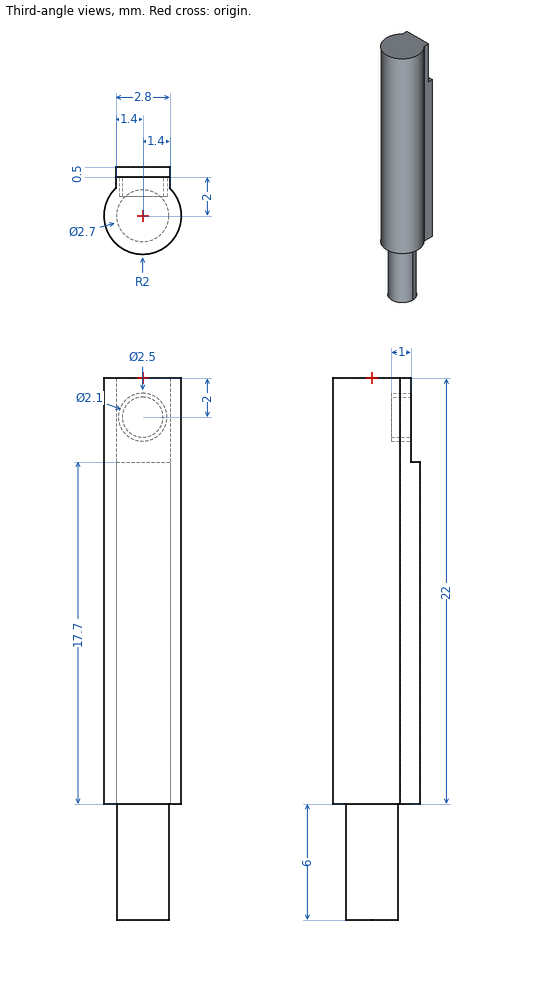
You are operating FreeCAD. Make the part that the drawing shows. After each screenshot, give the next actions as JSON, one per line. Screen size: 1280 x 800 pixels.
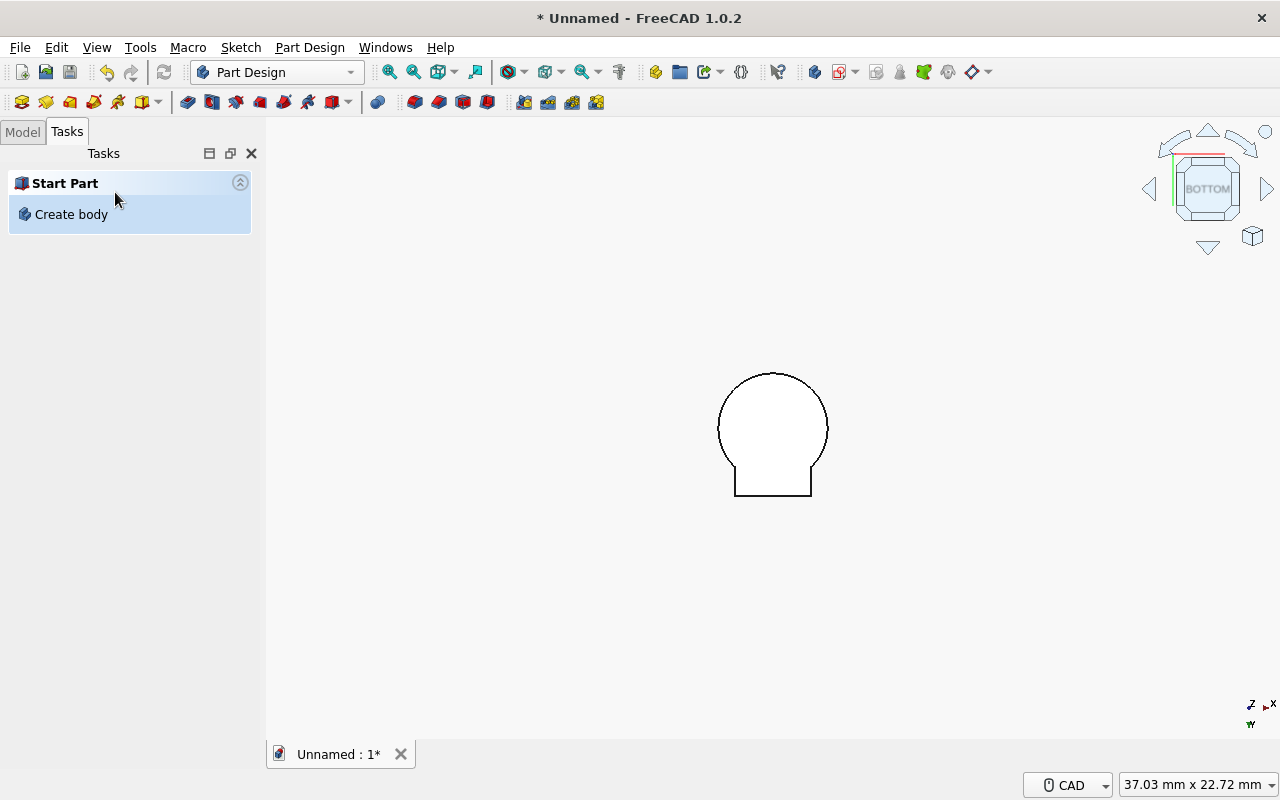
{"action": "left_click", "coordinate": [390, 72]}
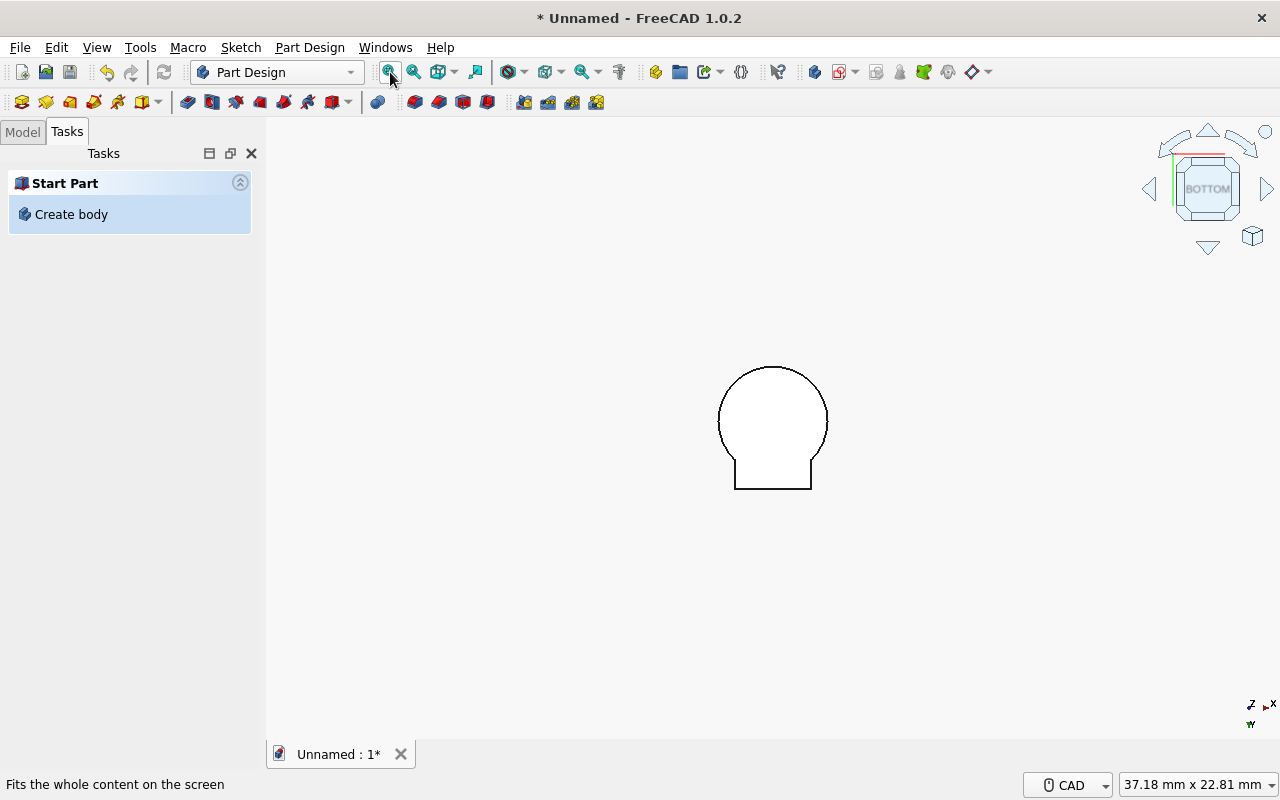
{"action": "key", "text": "4"}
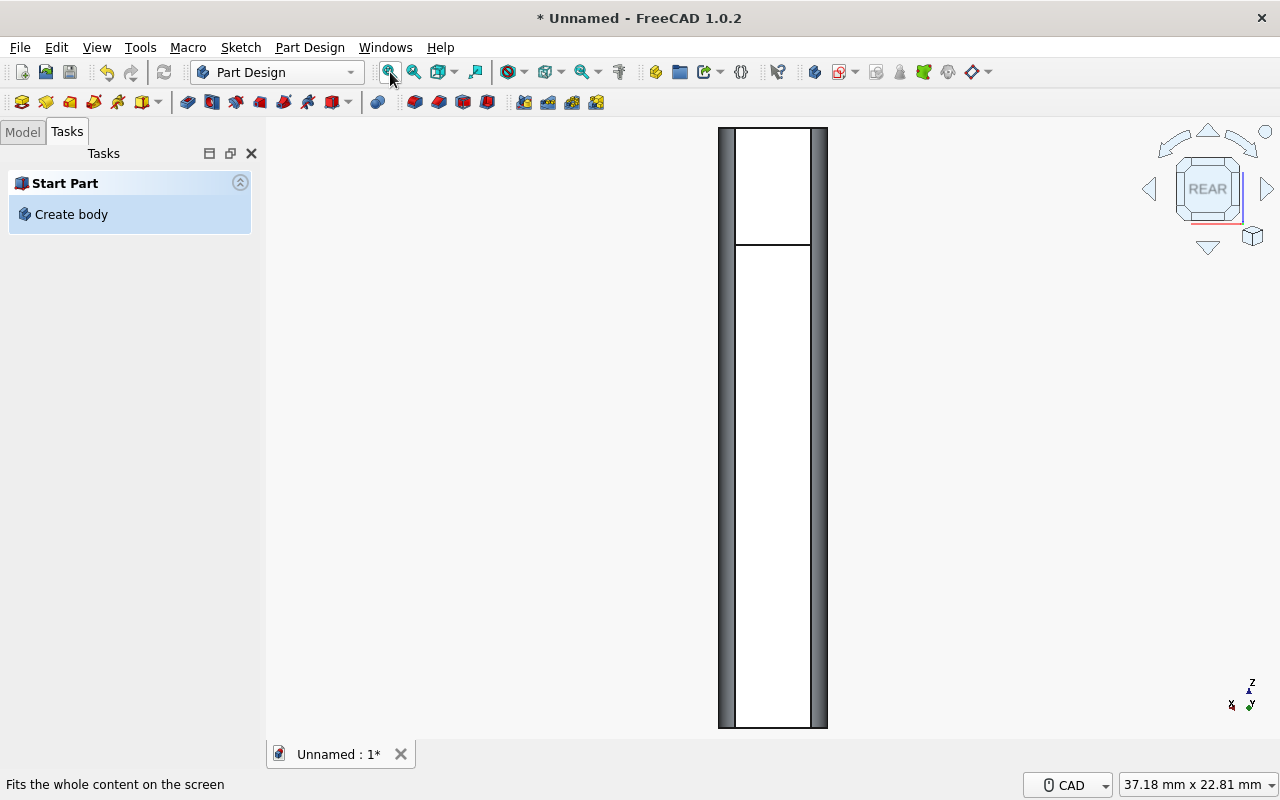
{"action": "left_click", "coordinate": [773, 169]}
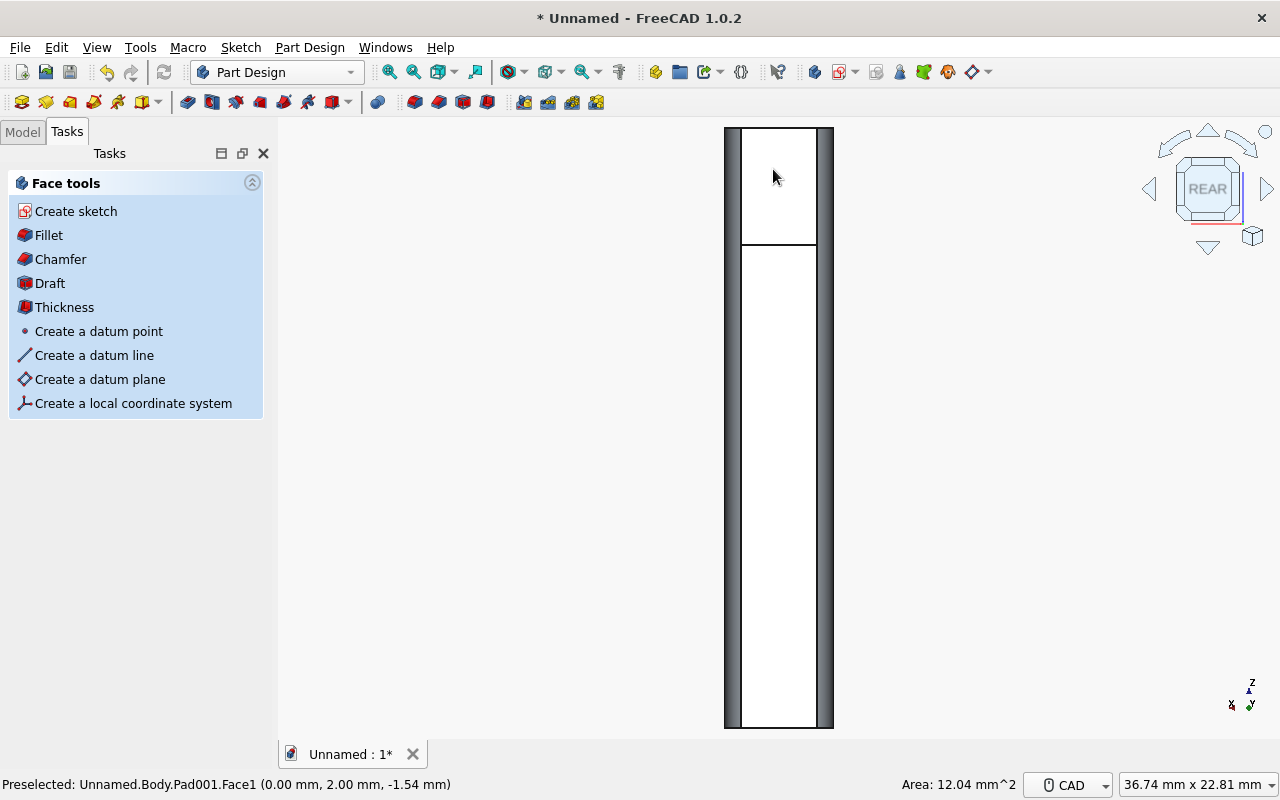
{"action": "left_click", "coordinate": [840, 72]}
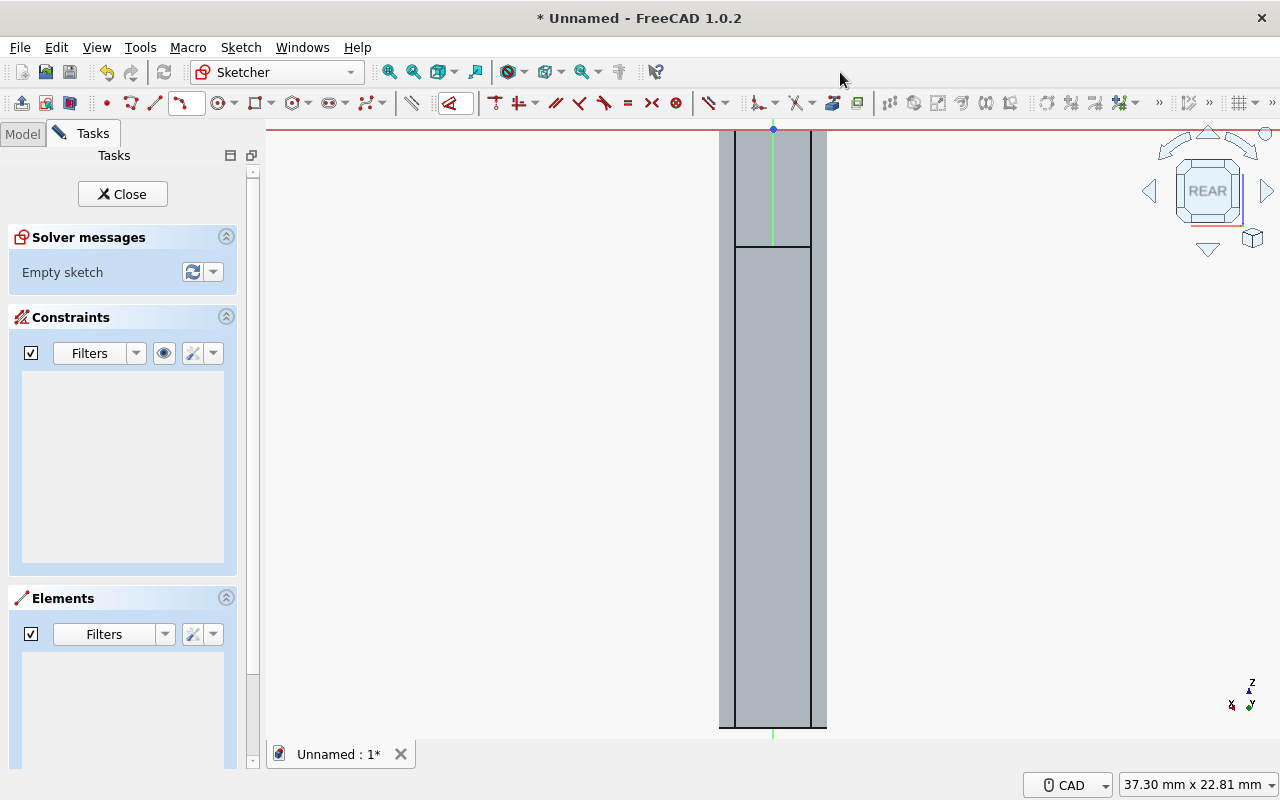
{"action": "left_click", "coordinate": [70, 104]}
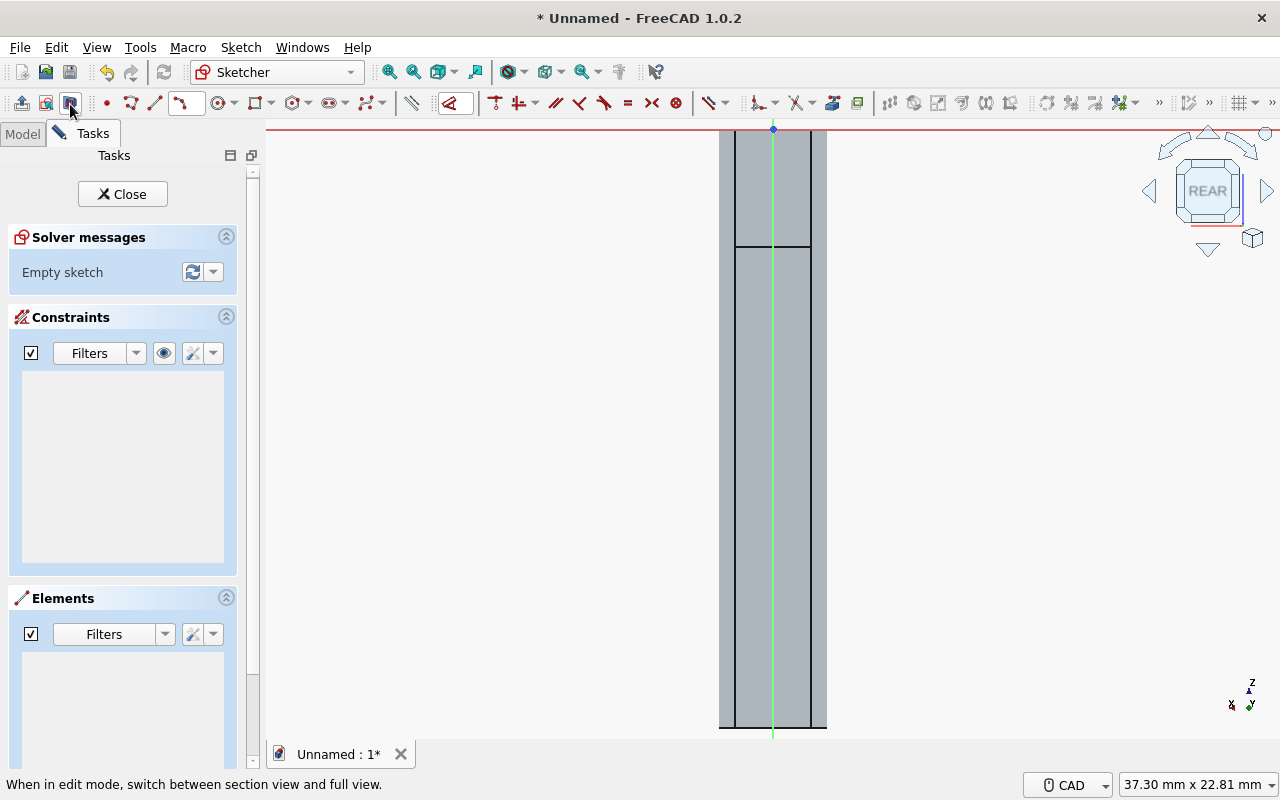
{"action": "scroll", "coordinate": [704, 429], "scroll_direction": "down", "scroll_amount": 5}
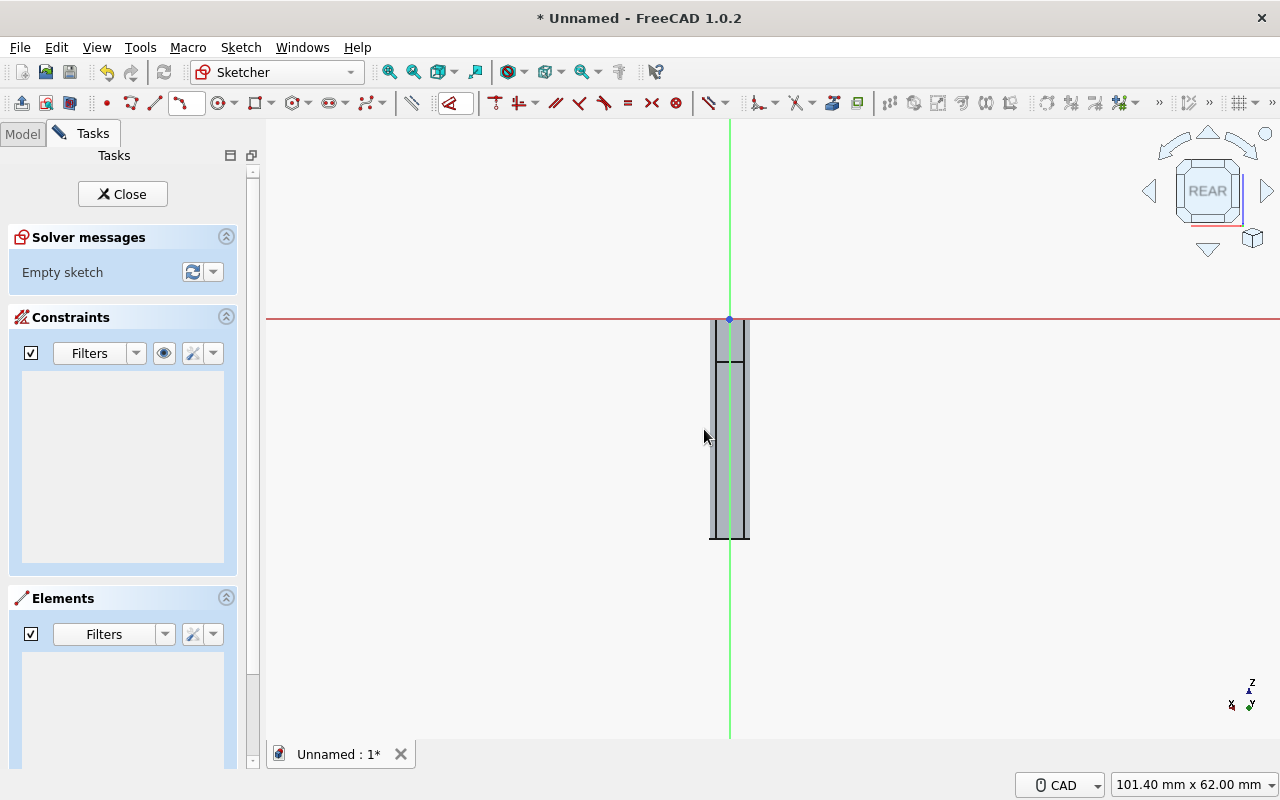
{"action": "scroll", "coordinate": [732, 328], "scroll_direction": "up", "scroll_amount": 13}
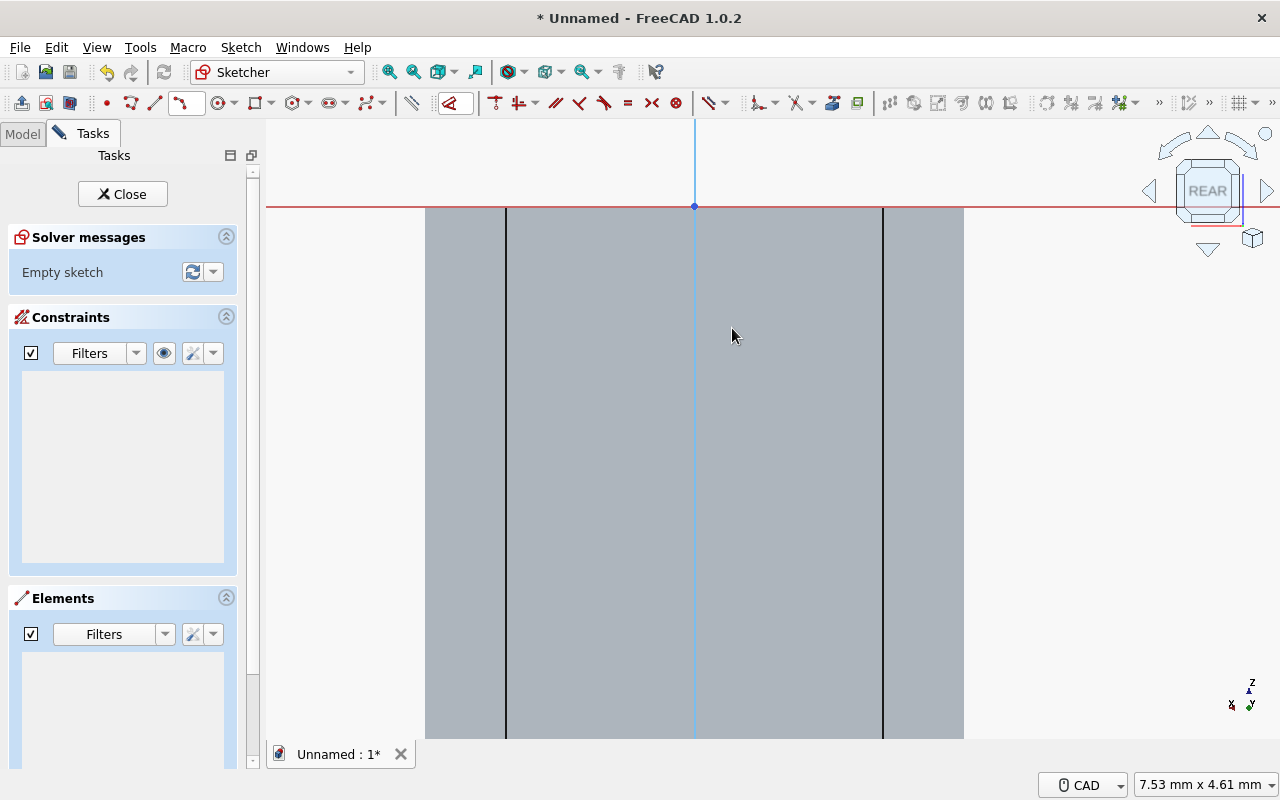
{"action": "left_click", "coordinate": [218, 104]}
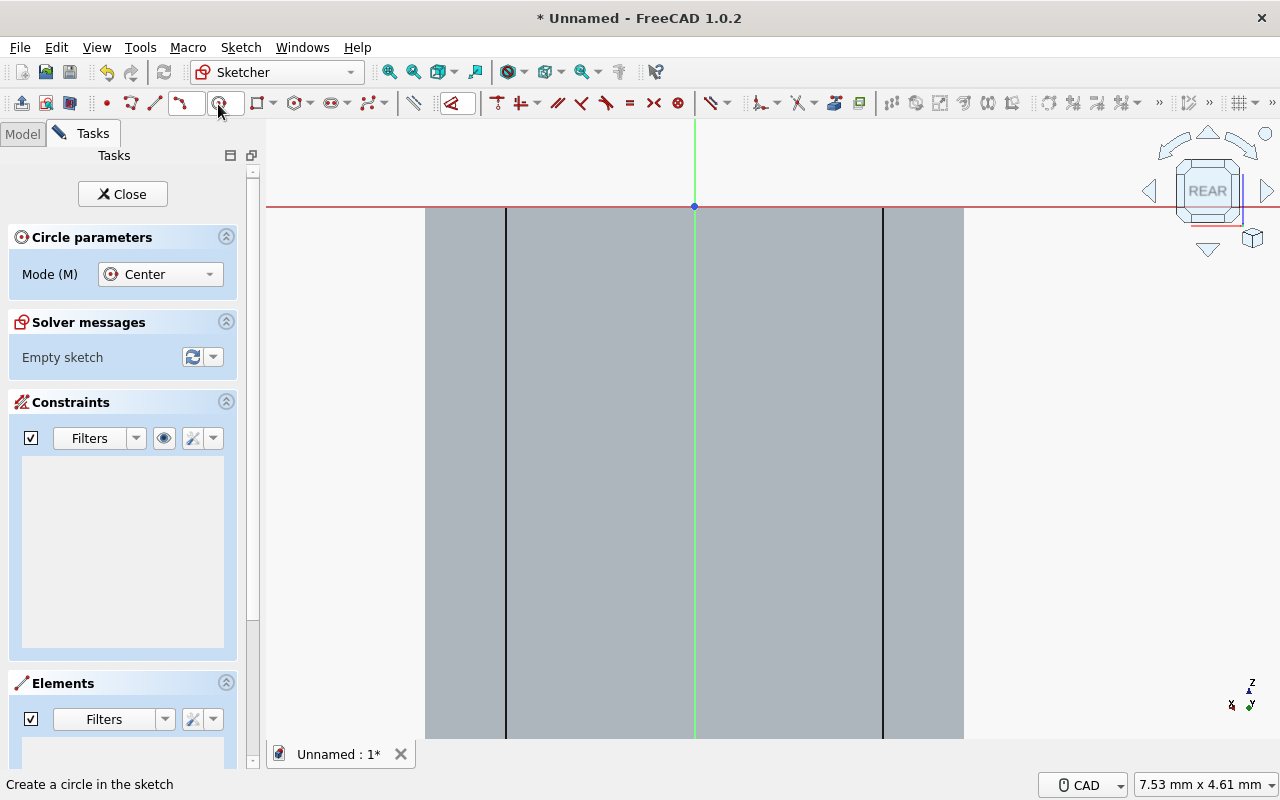
{"action": "left_click", "coordinate": [695, 476]}
{"action": "left_click", "coordinate": [814, 357]}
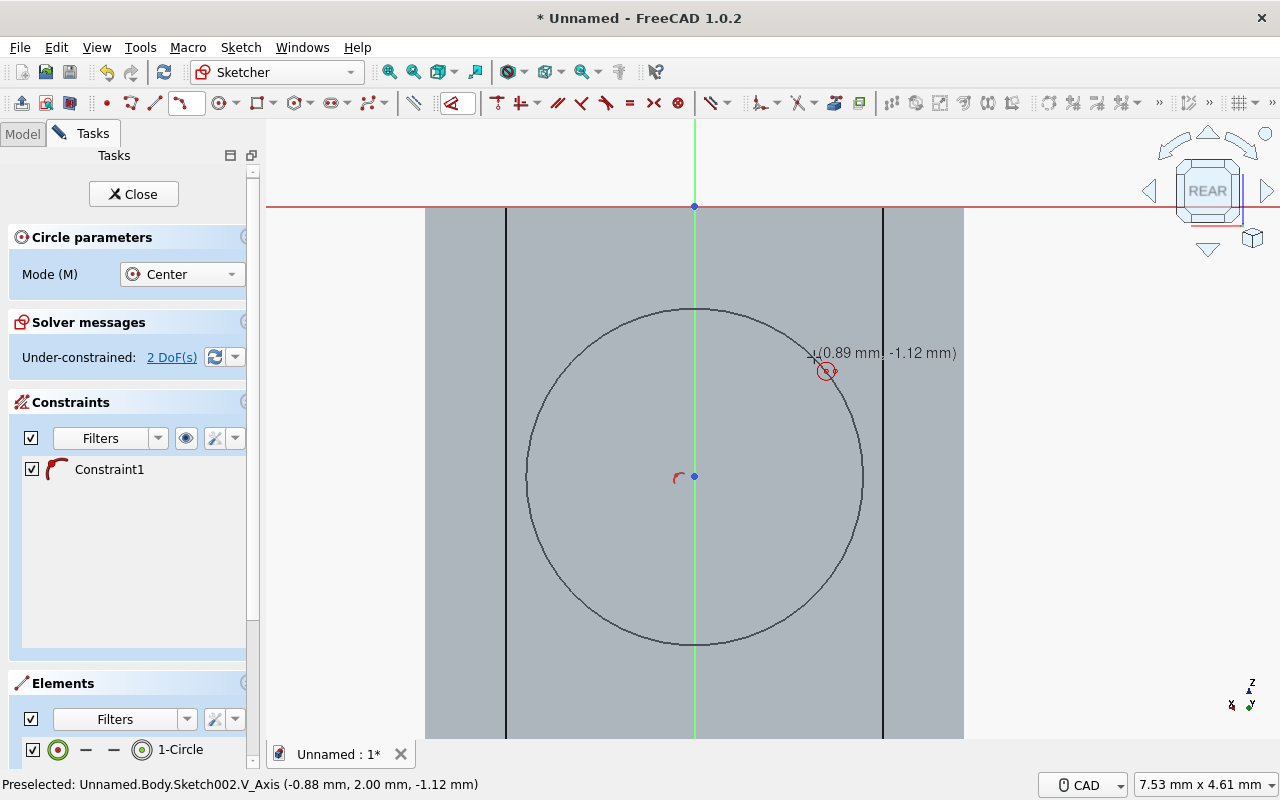
{"action": "left_click", "coordinate": [695, 477]}
{"action": "left_click", "coordinate": [795, 376]}
{"action": "key", "text": "Escape"}